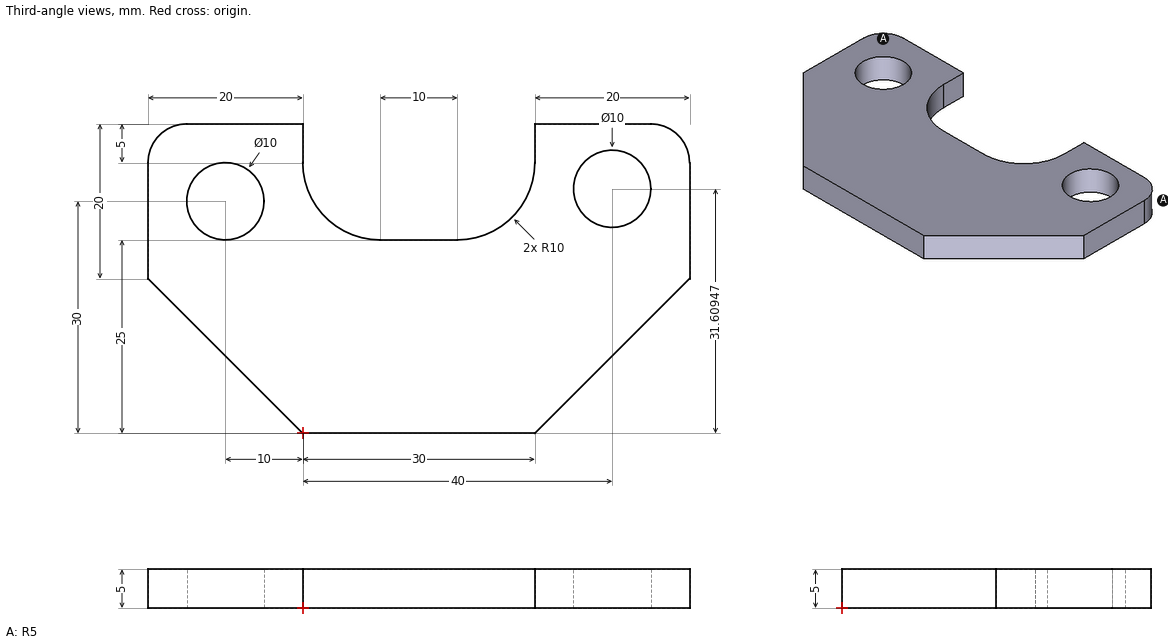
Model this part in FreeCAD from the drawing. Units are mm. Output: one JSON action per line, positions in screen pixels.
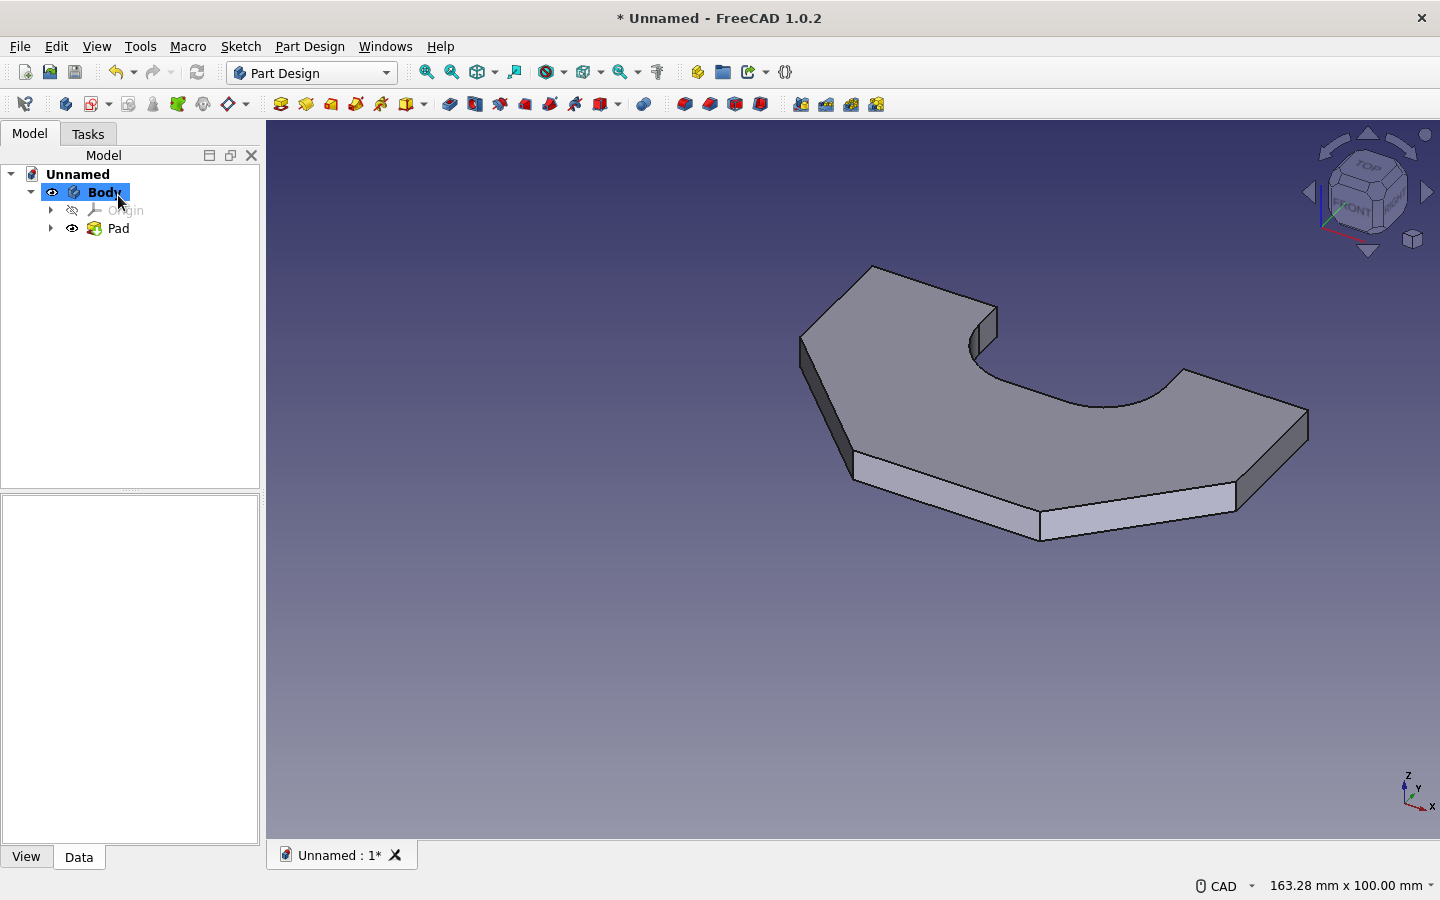
{"action": "left_click", "coordinate": [1060, 450]}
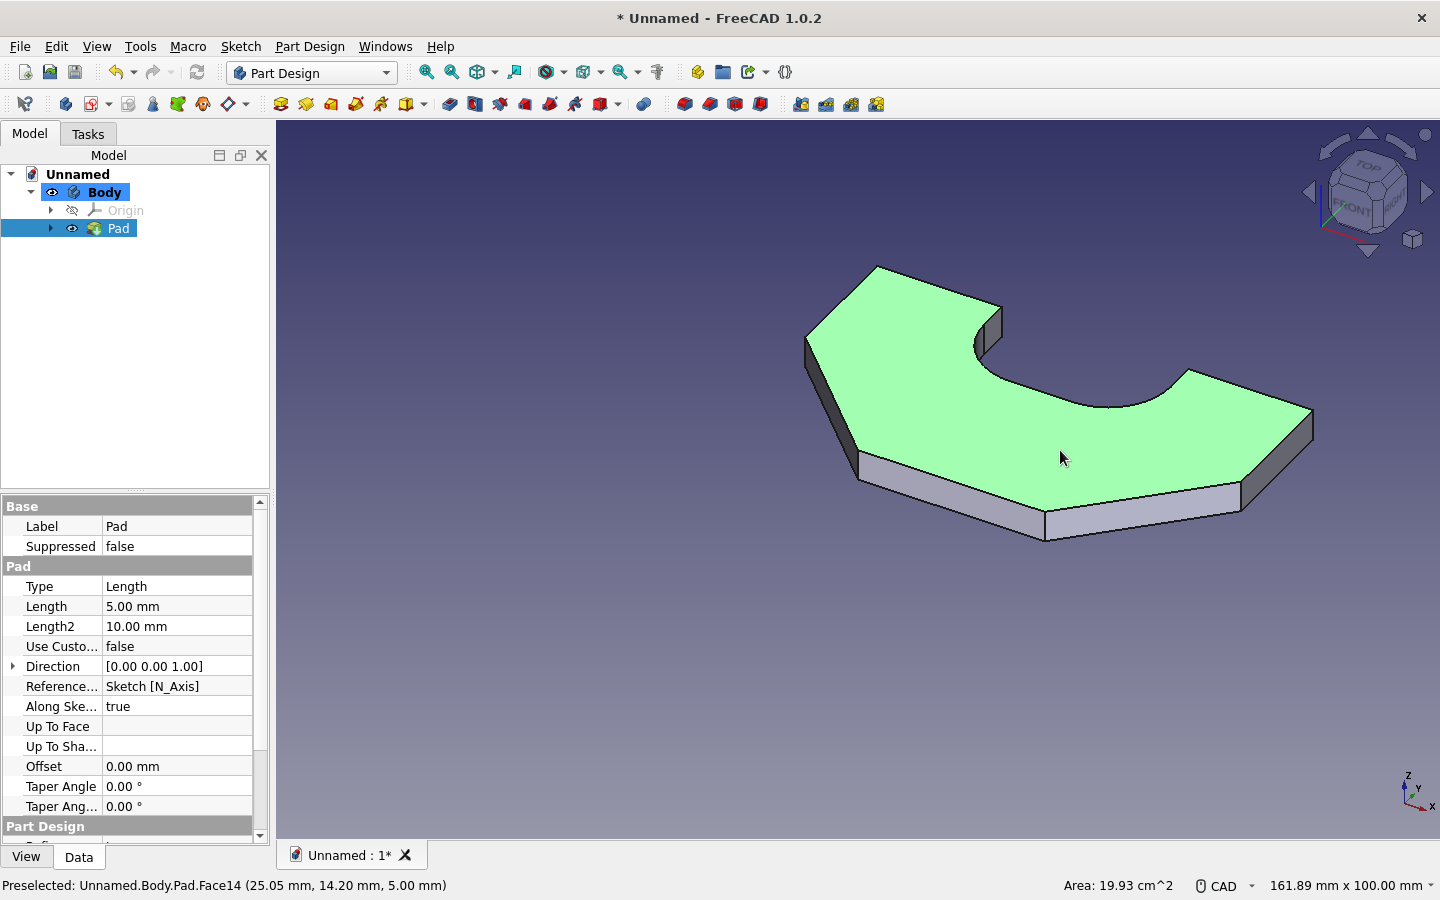
{"action": "left_click", "coordinate": [90, 104]}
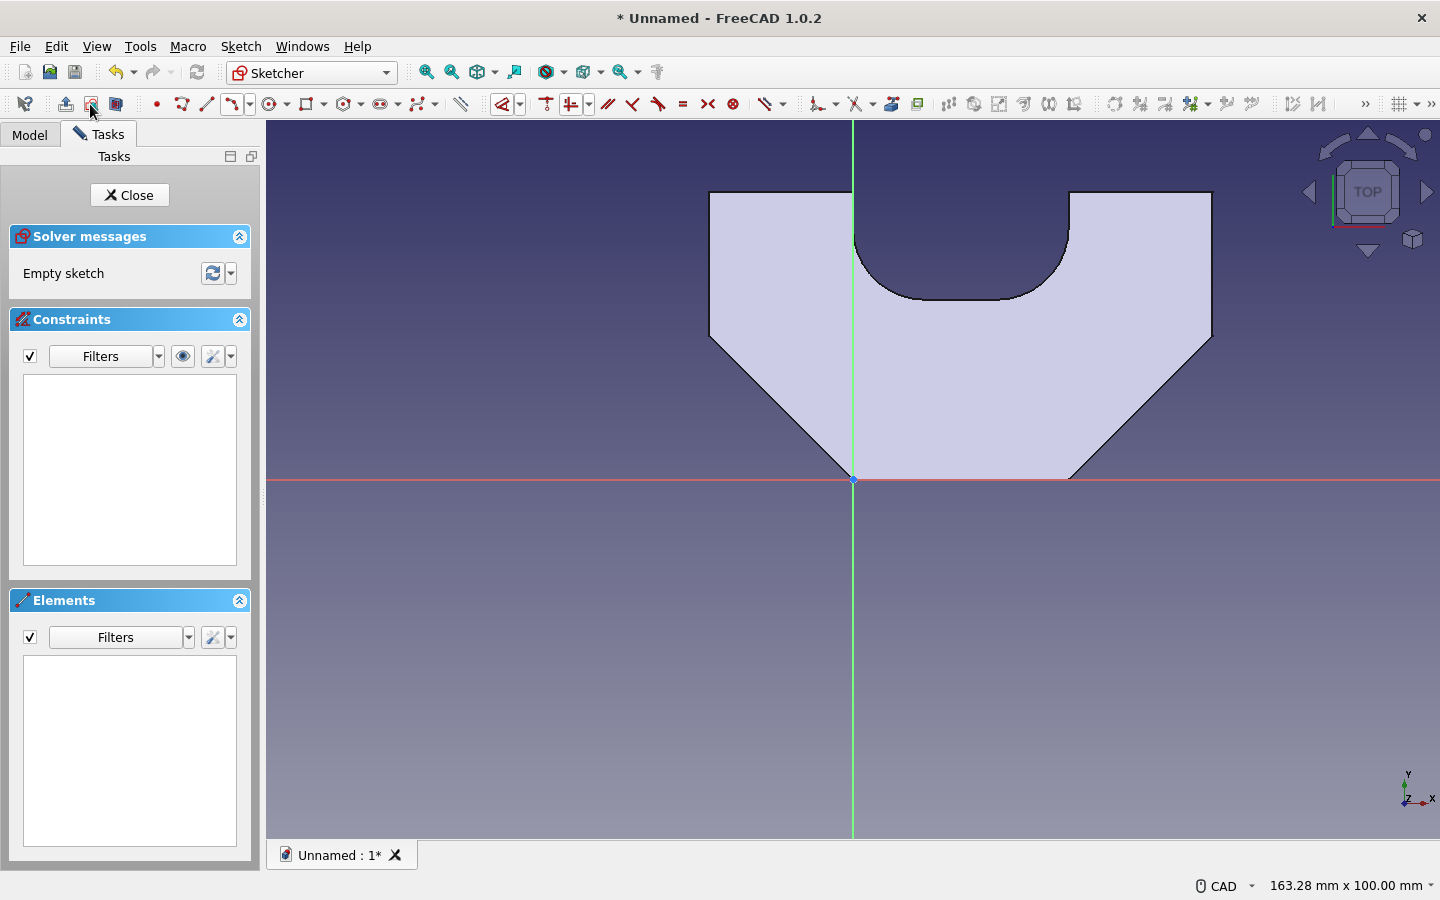
{"action": "scroll", "coordinate": [780, 221], "scroll_direction": "up", "scroll_amount": 9}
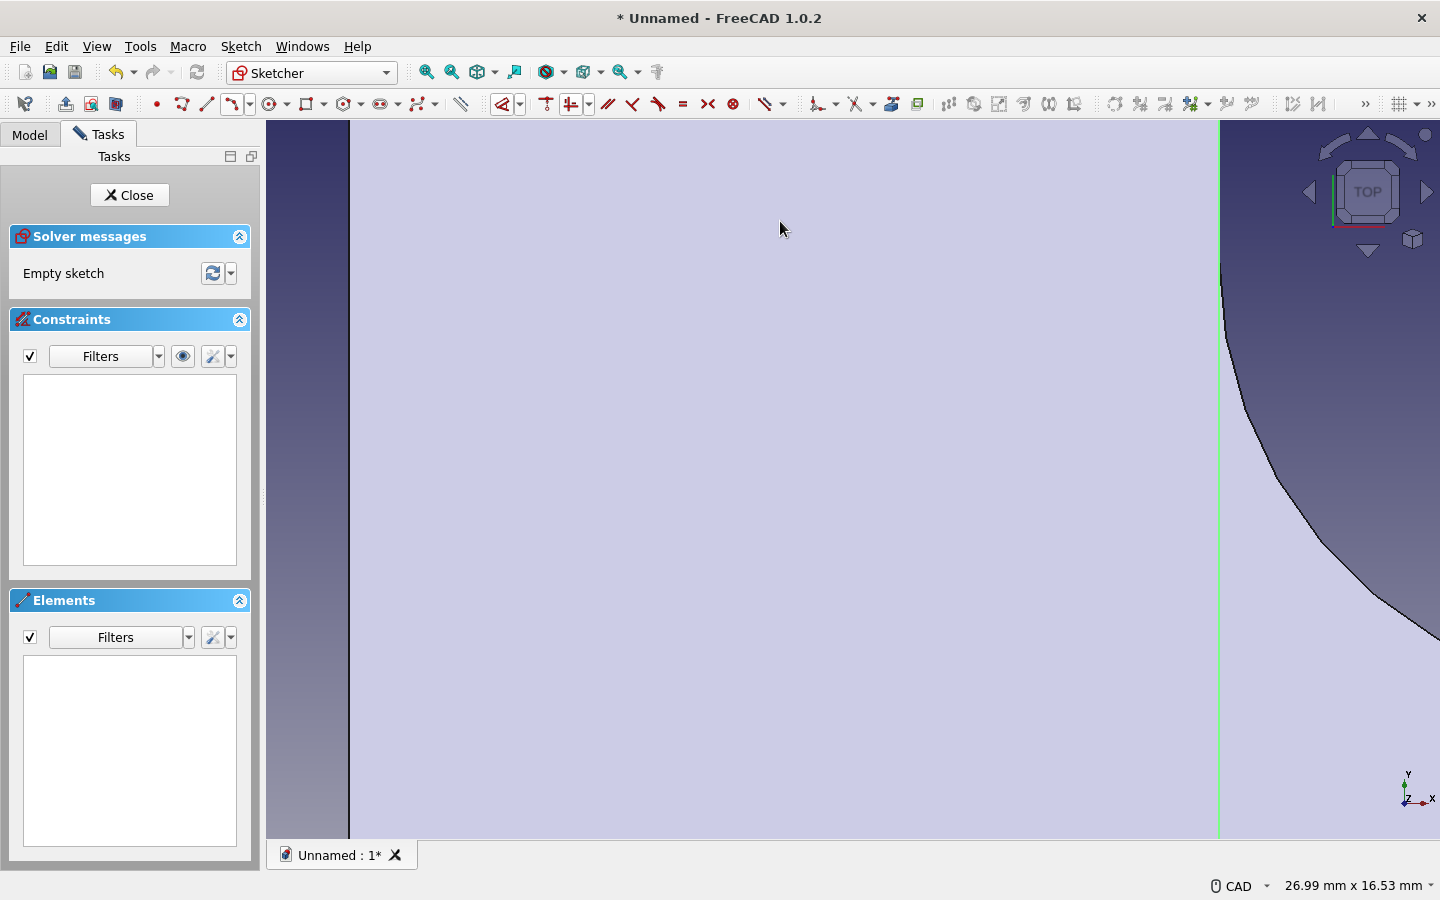
{"action": "left_click", "coordinate": [268, 104]}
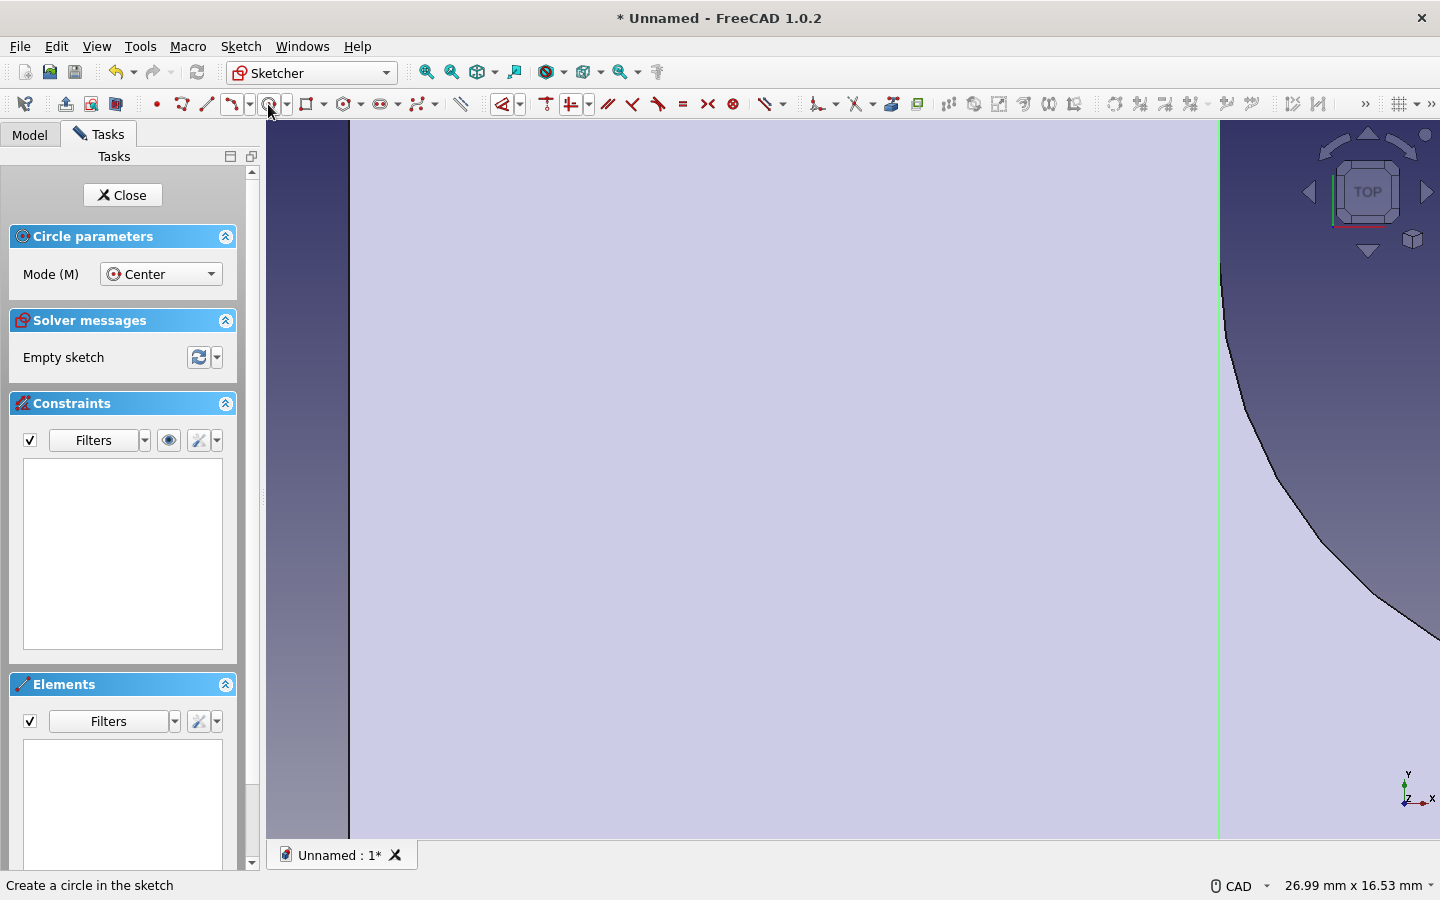
{"action": "left_click", "coordinate": [784, 479]}
{"action": "left_click", "coordinate": [938, 325]}
{"action": "key", "text": "Escape"}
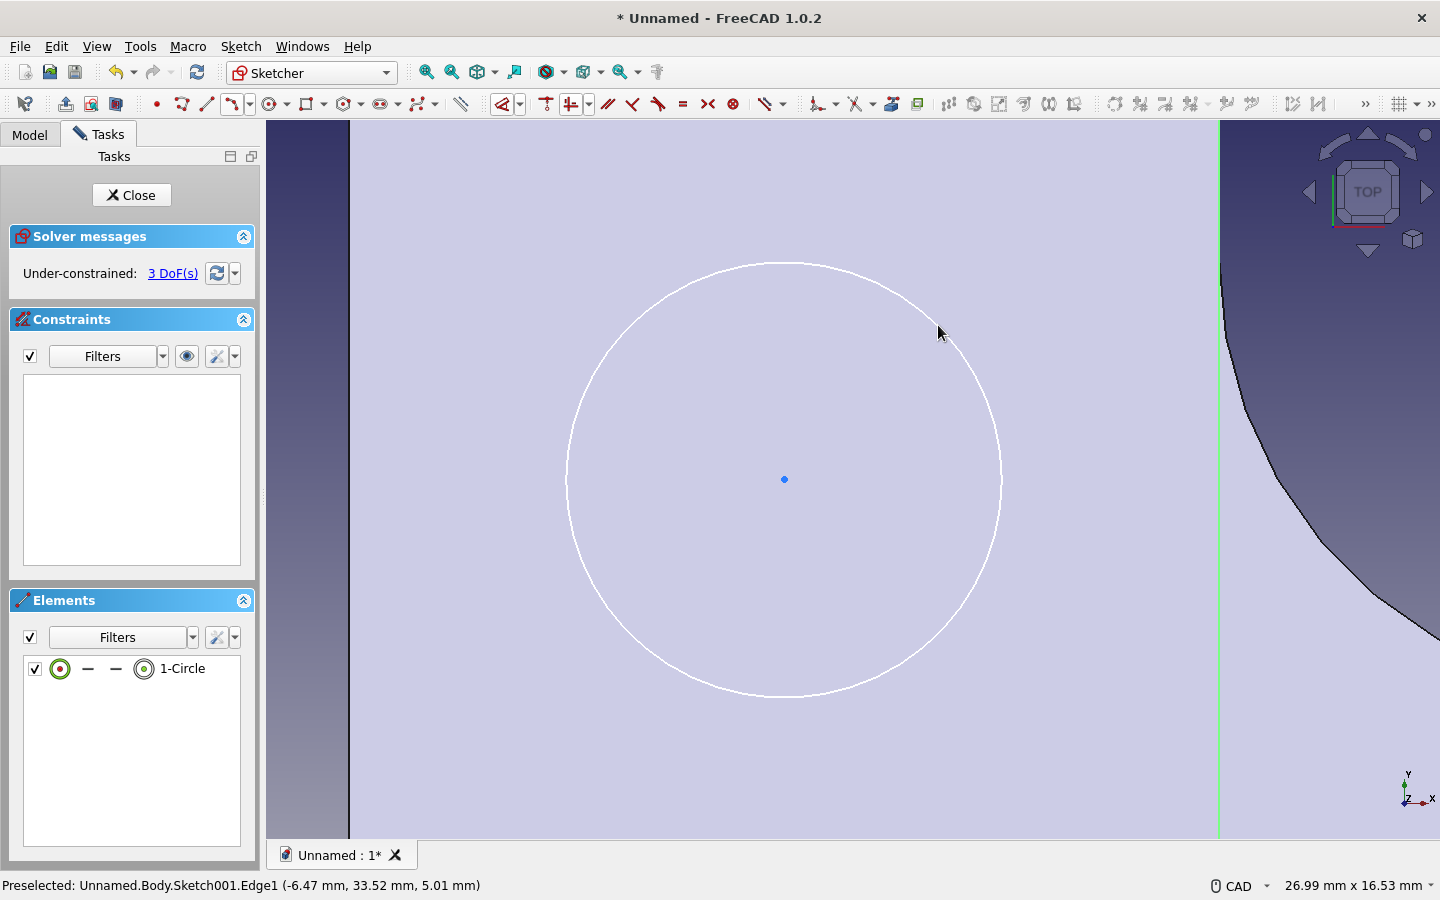
{"action": "left_click", "coordinate": [938, 326]}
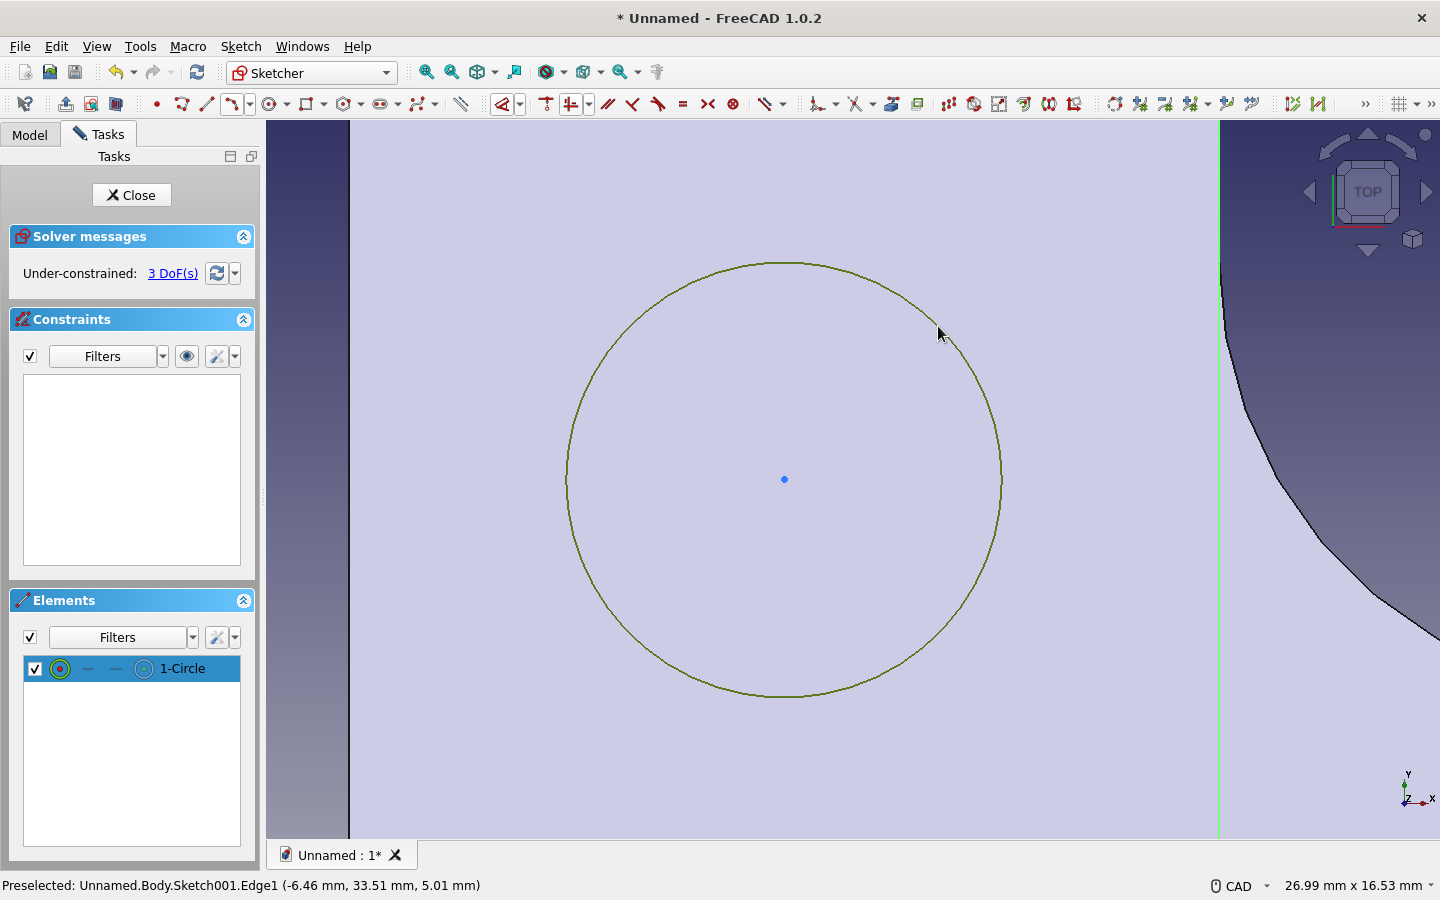
{"action": "left_click", "coordinate": [520, 104]}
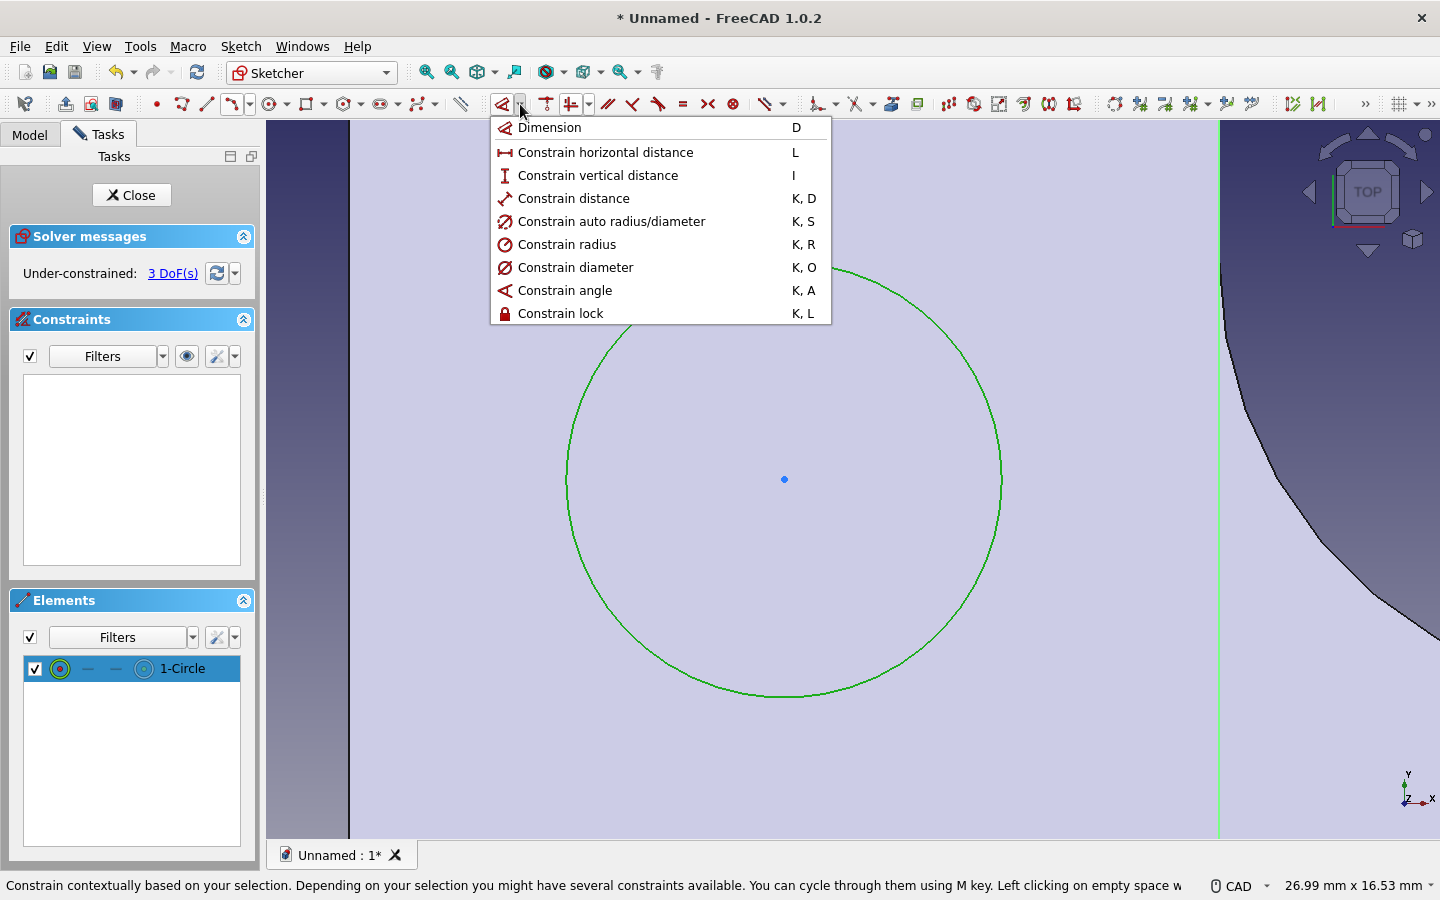
{"action": "left_click", "coordinate": [661, 268]}